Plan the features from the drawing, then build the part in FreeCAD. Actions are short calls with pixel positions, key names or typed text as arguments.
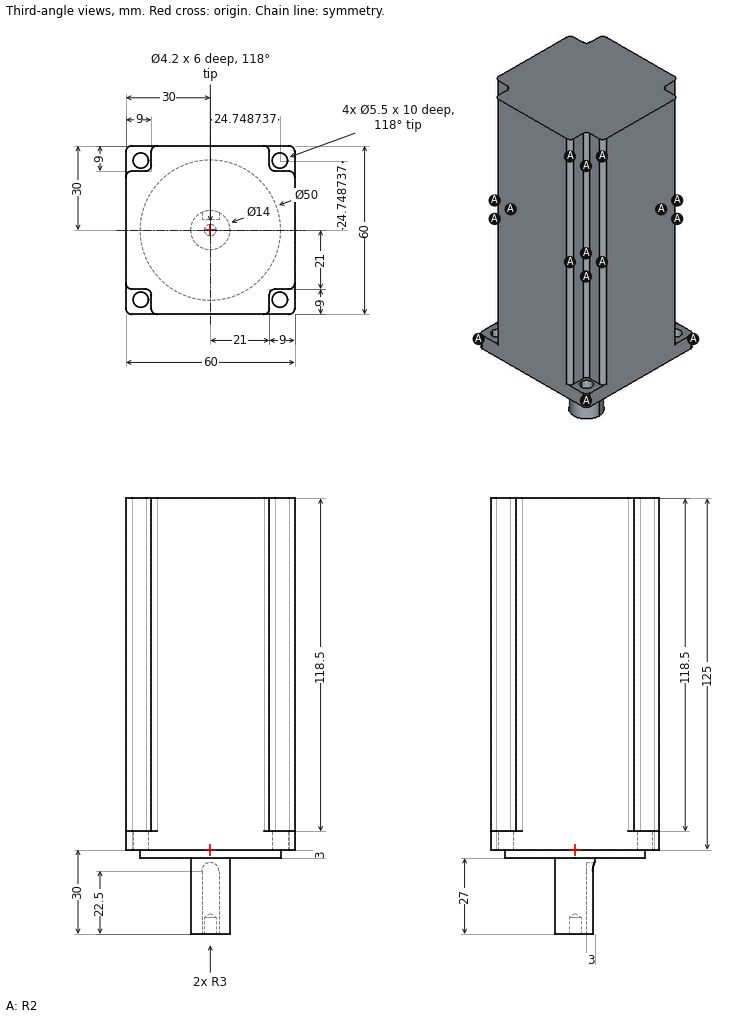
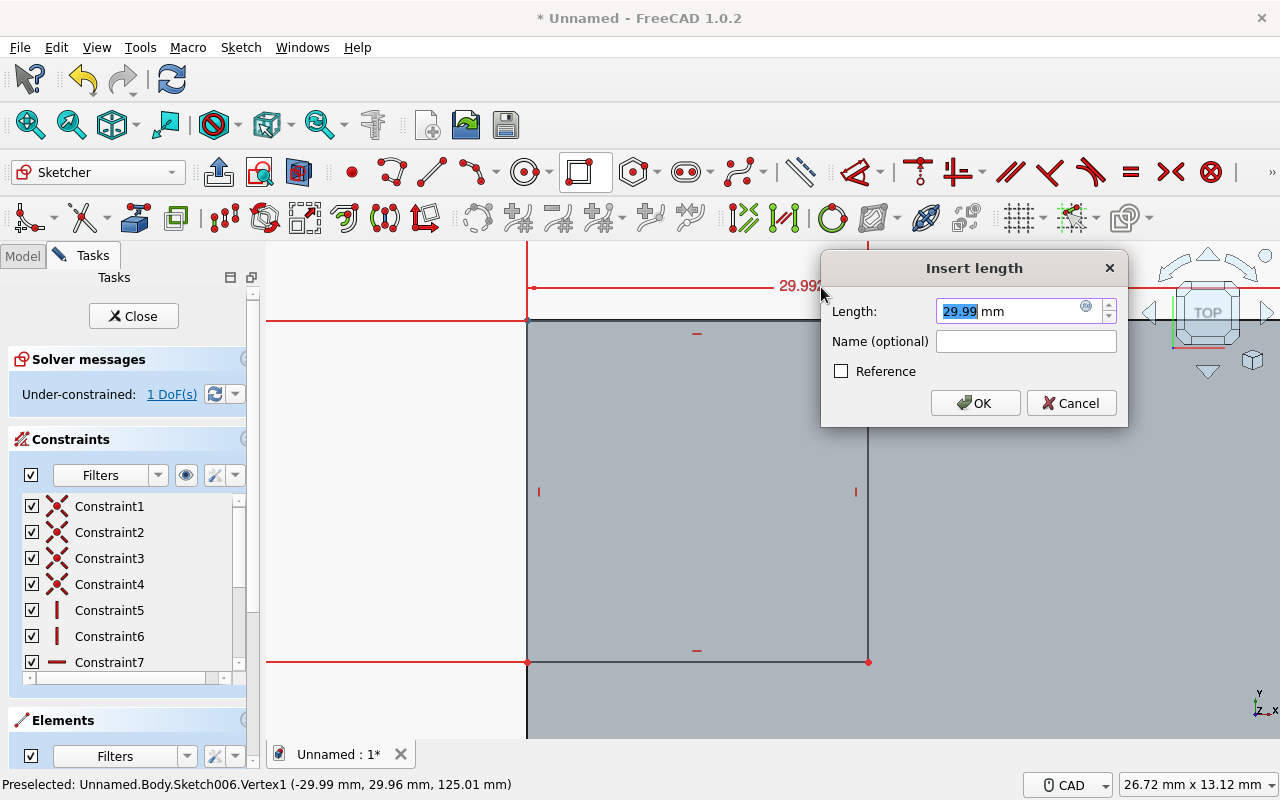
text(30)
key(Return)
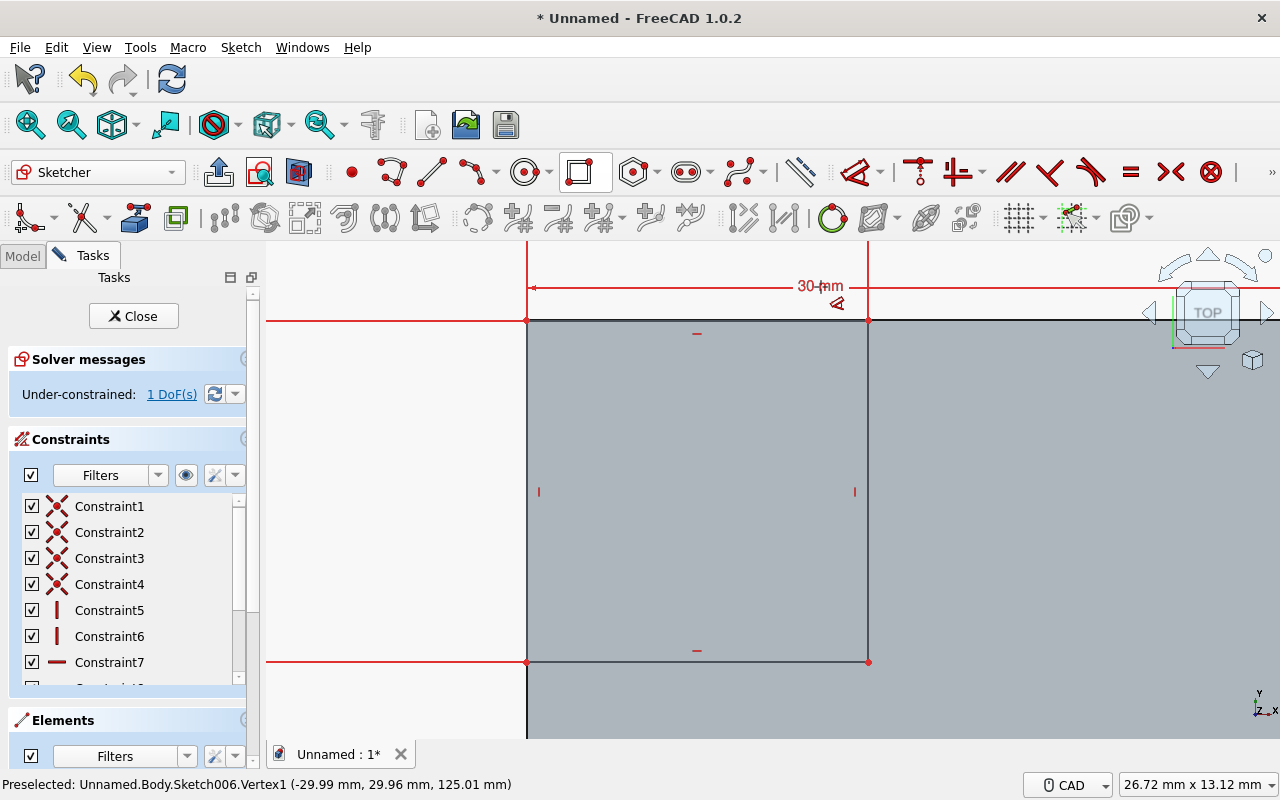
click(527, 321)
click(493, 516)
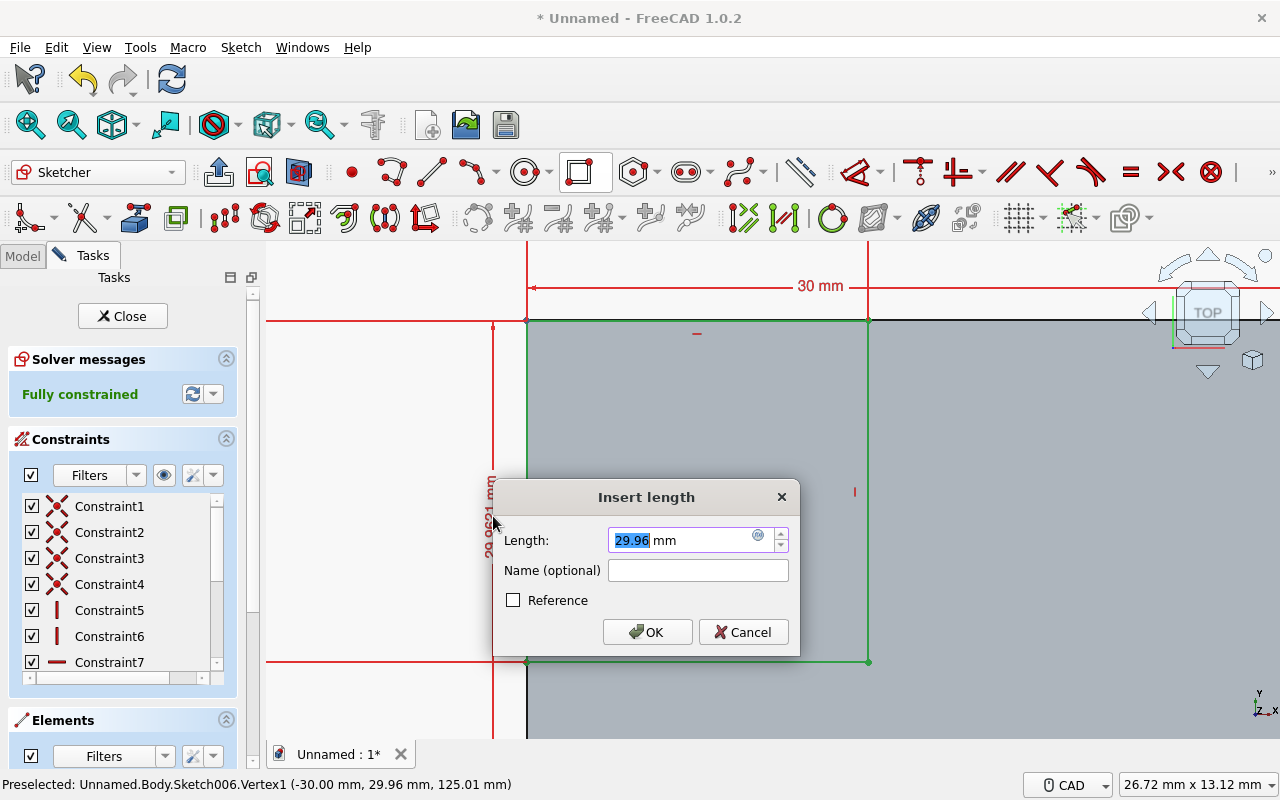
text(30)
key(Return)
key(Escape)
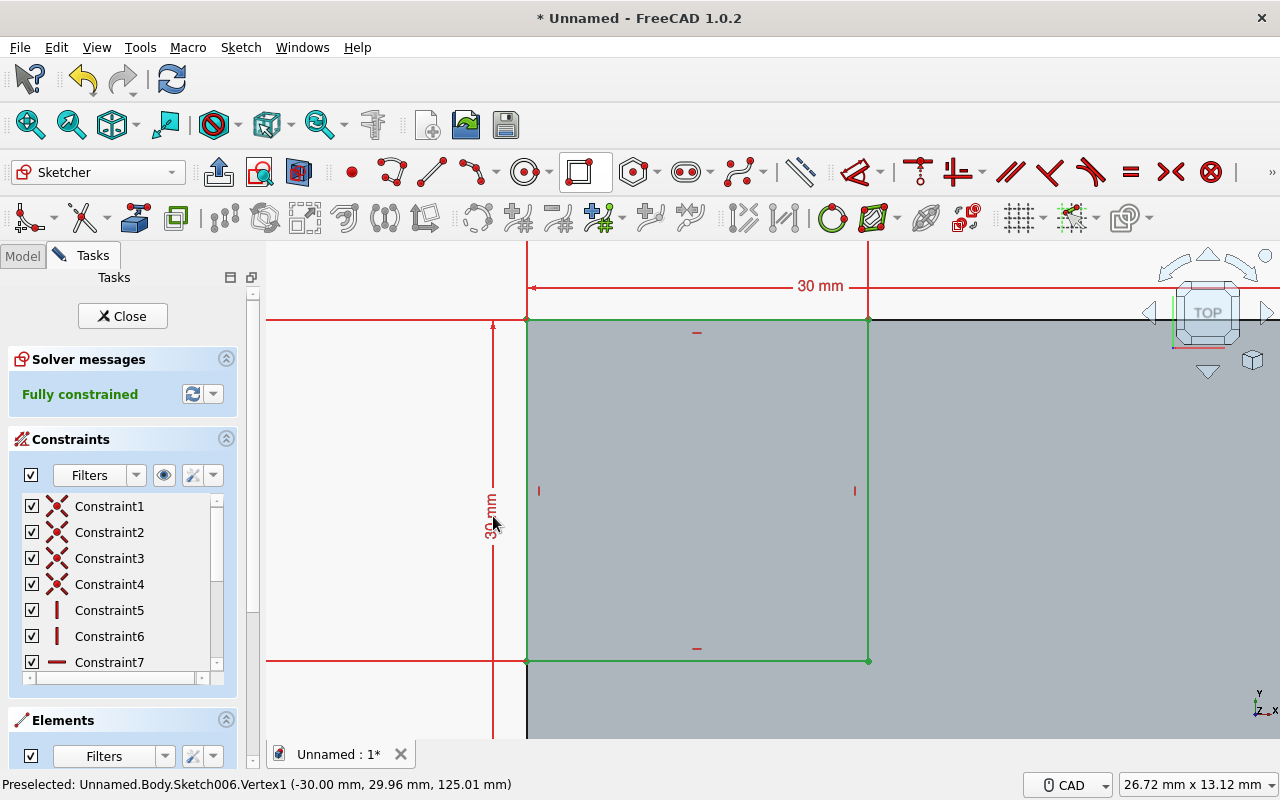
click(123, 316)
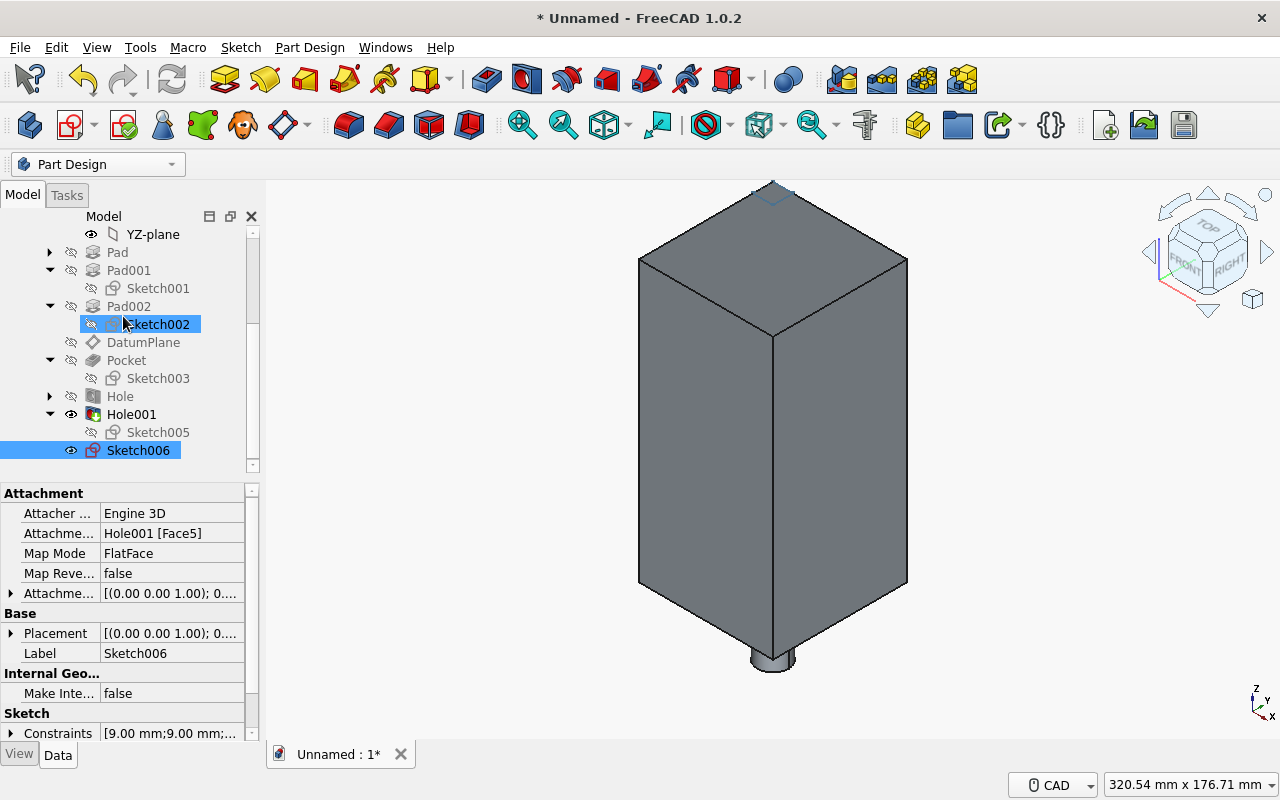
click(488, 80)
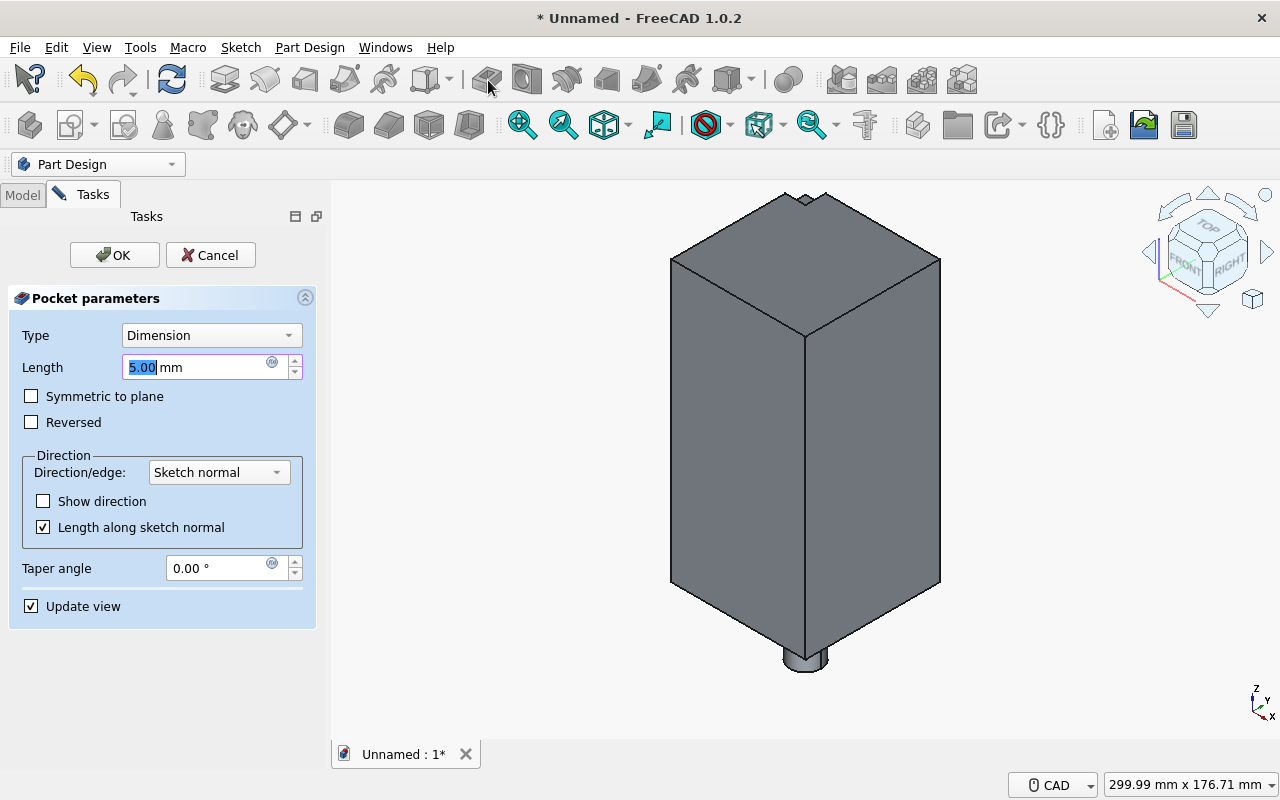
text(118.5)
key(Tab)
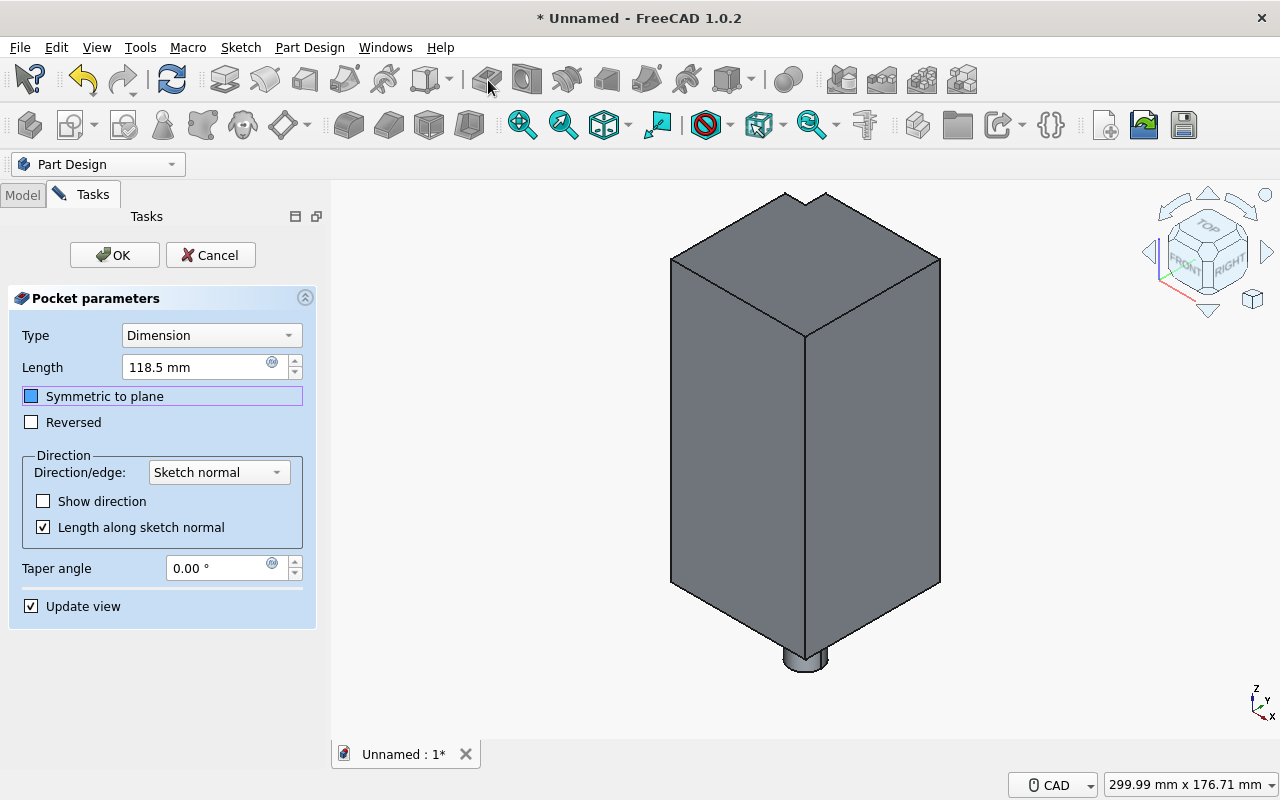
click(115, 255)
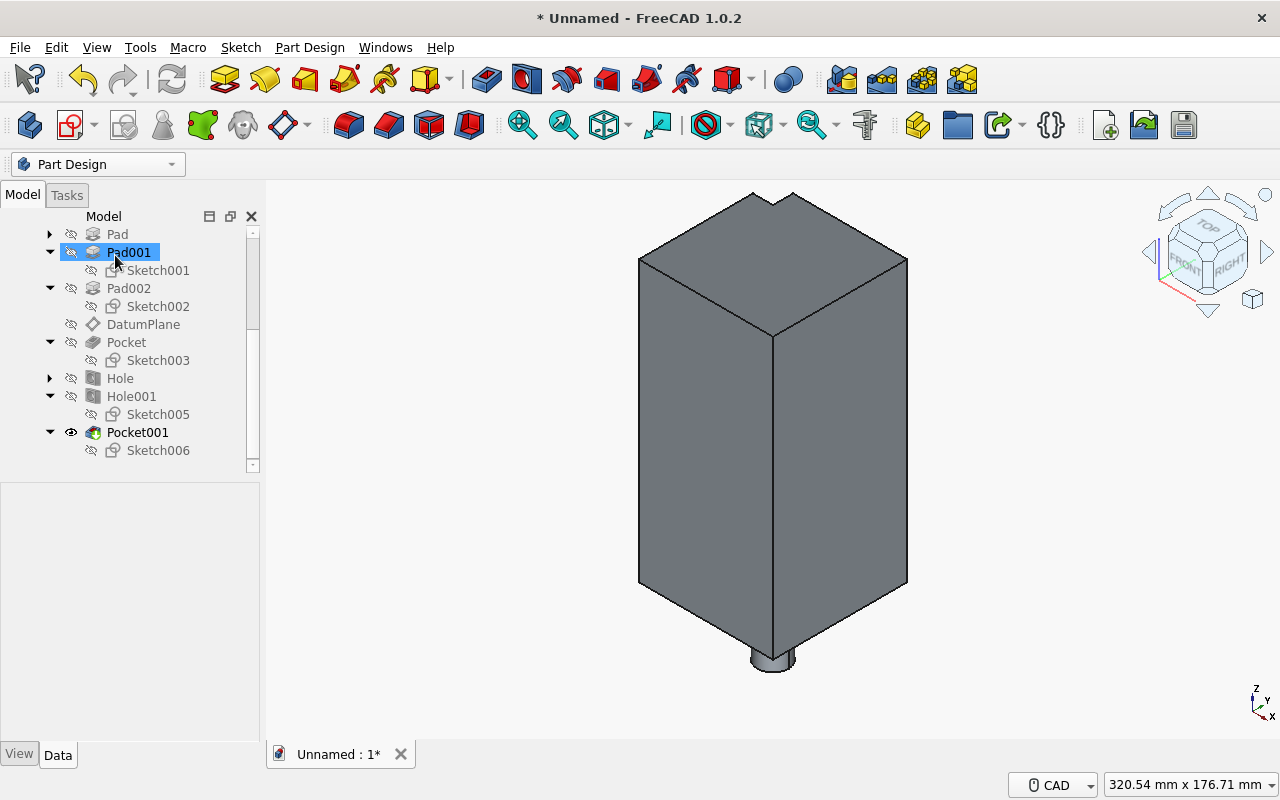
click(116, 432)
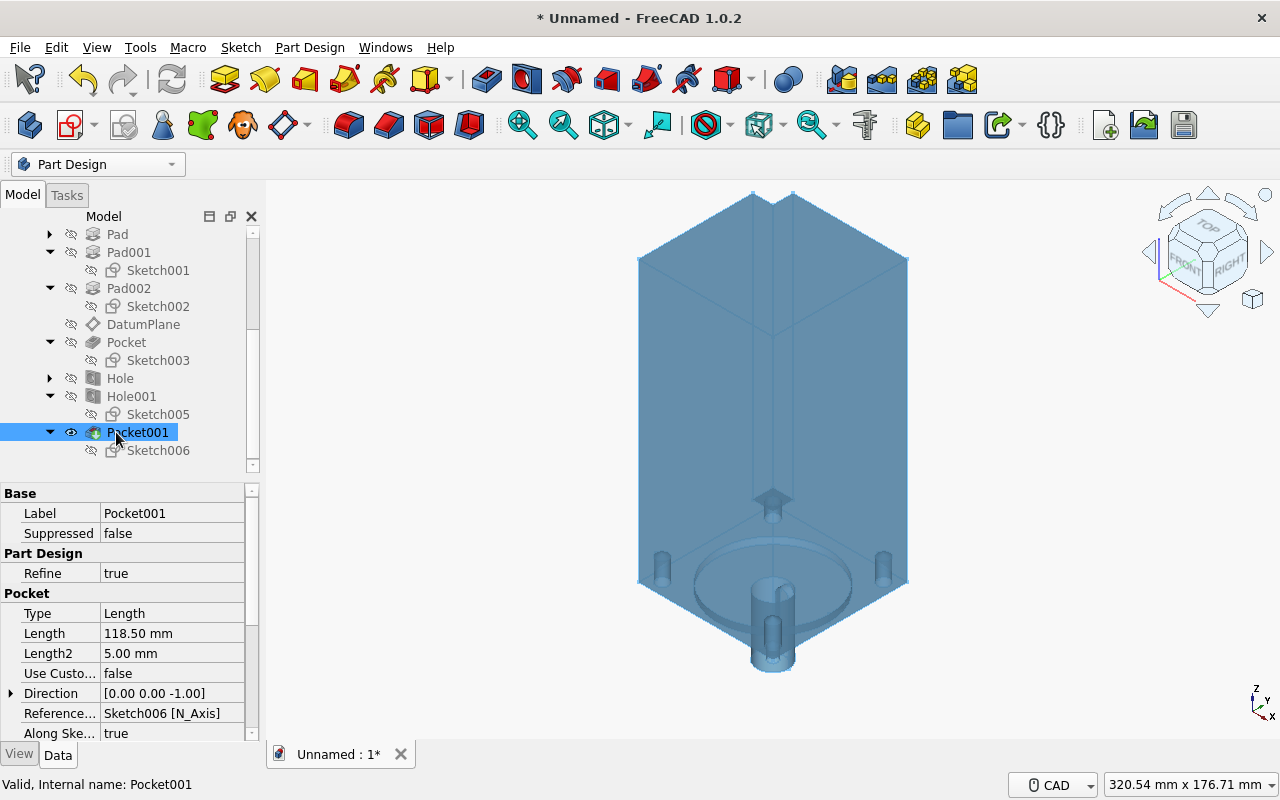
click(842, 80)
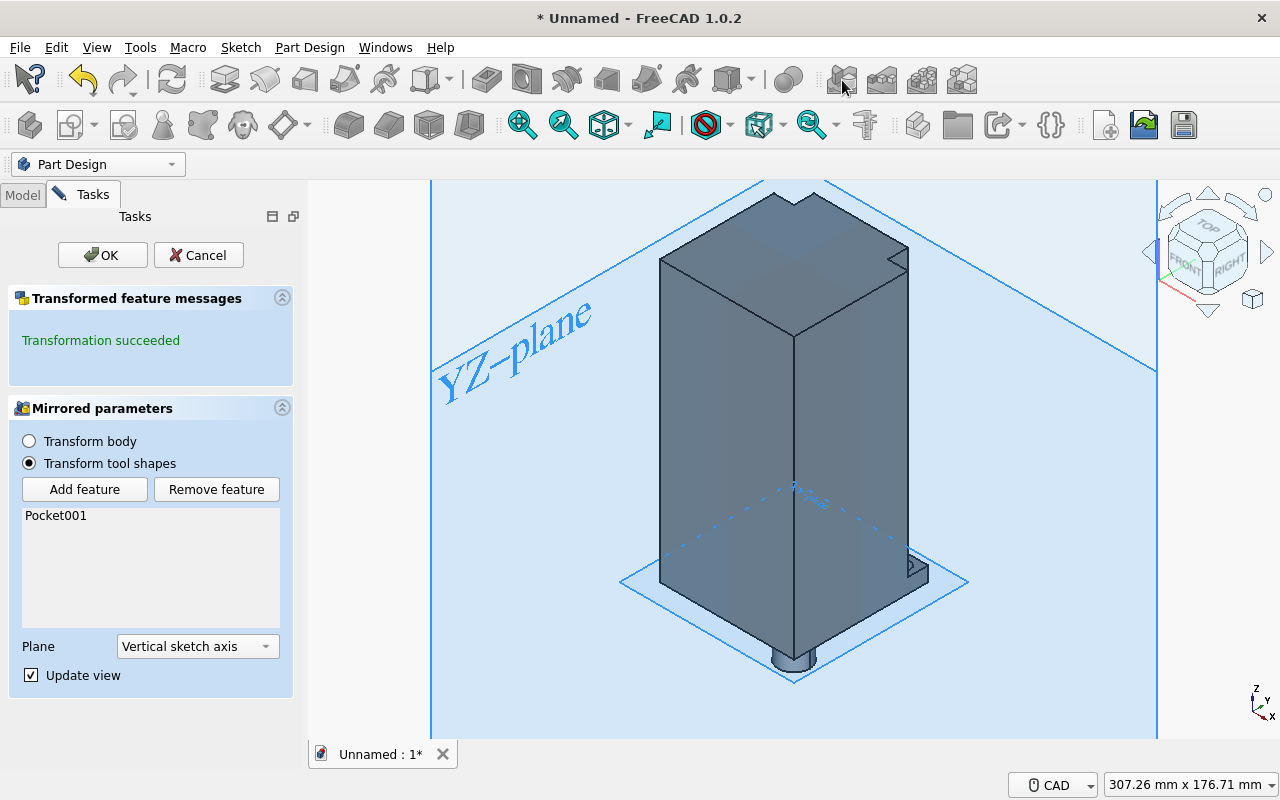
click(198, 646)